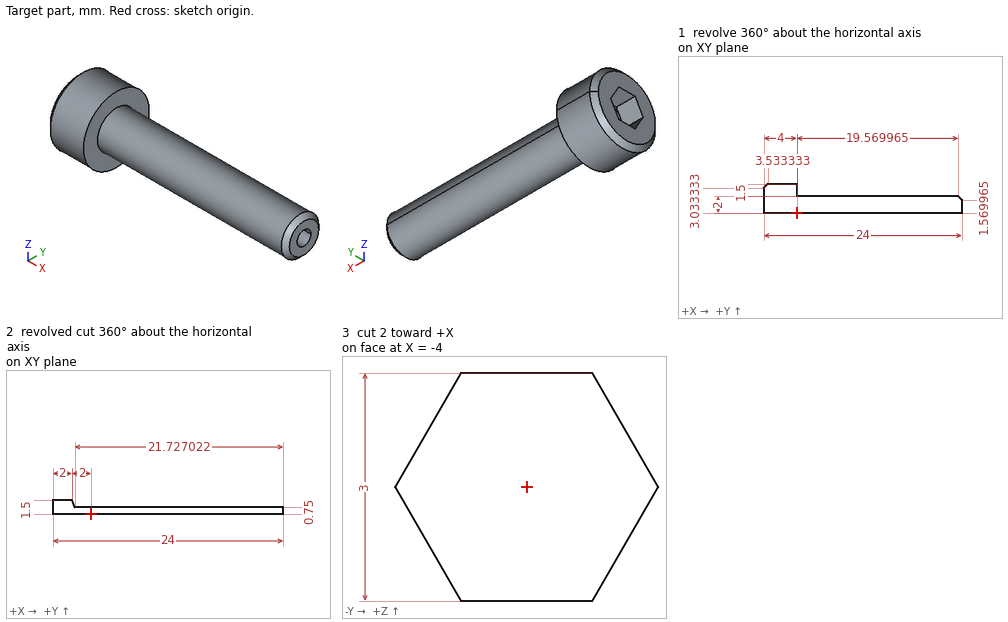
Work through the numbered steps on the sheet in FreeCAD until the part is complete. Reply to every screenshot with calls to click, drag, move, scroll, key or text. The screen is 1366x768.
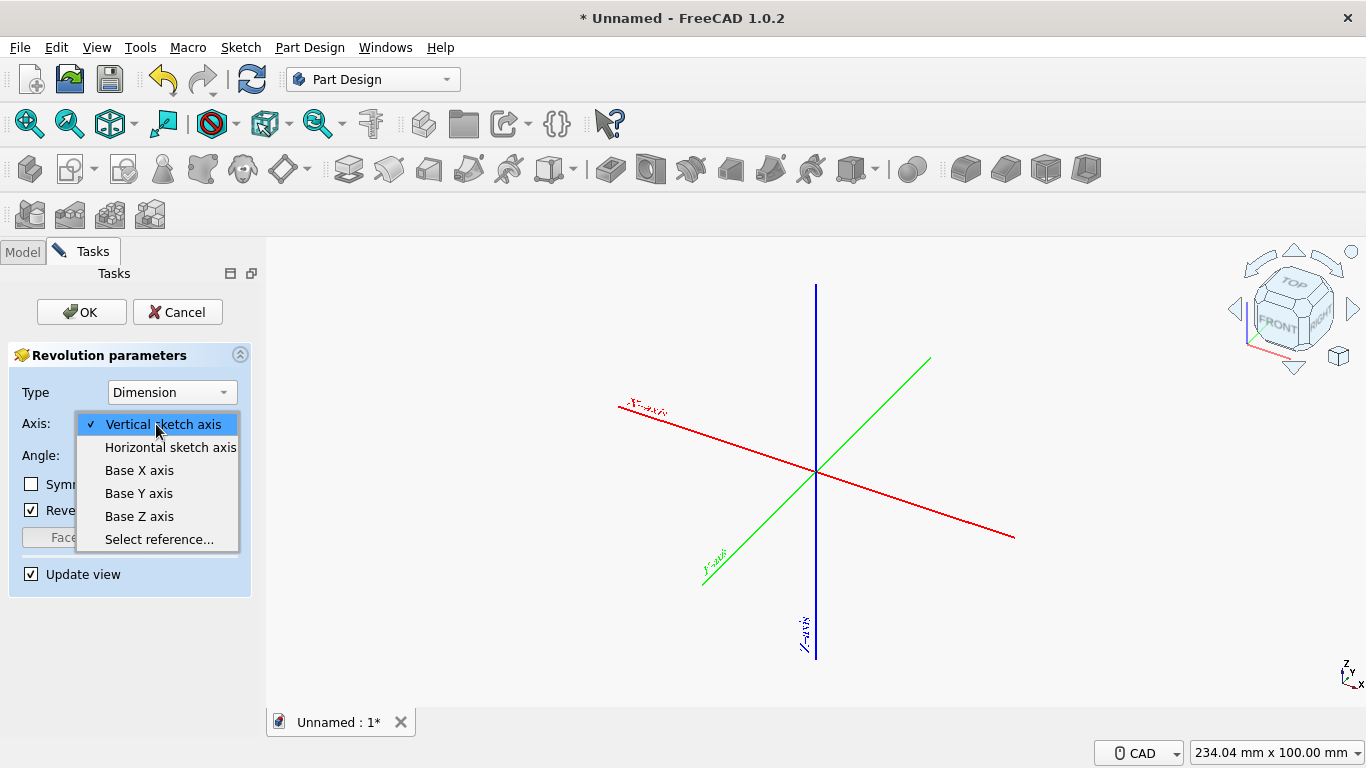
click(156, 448)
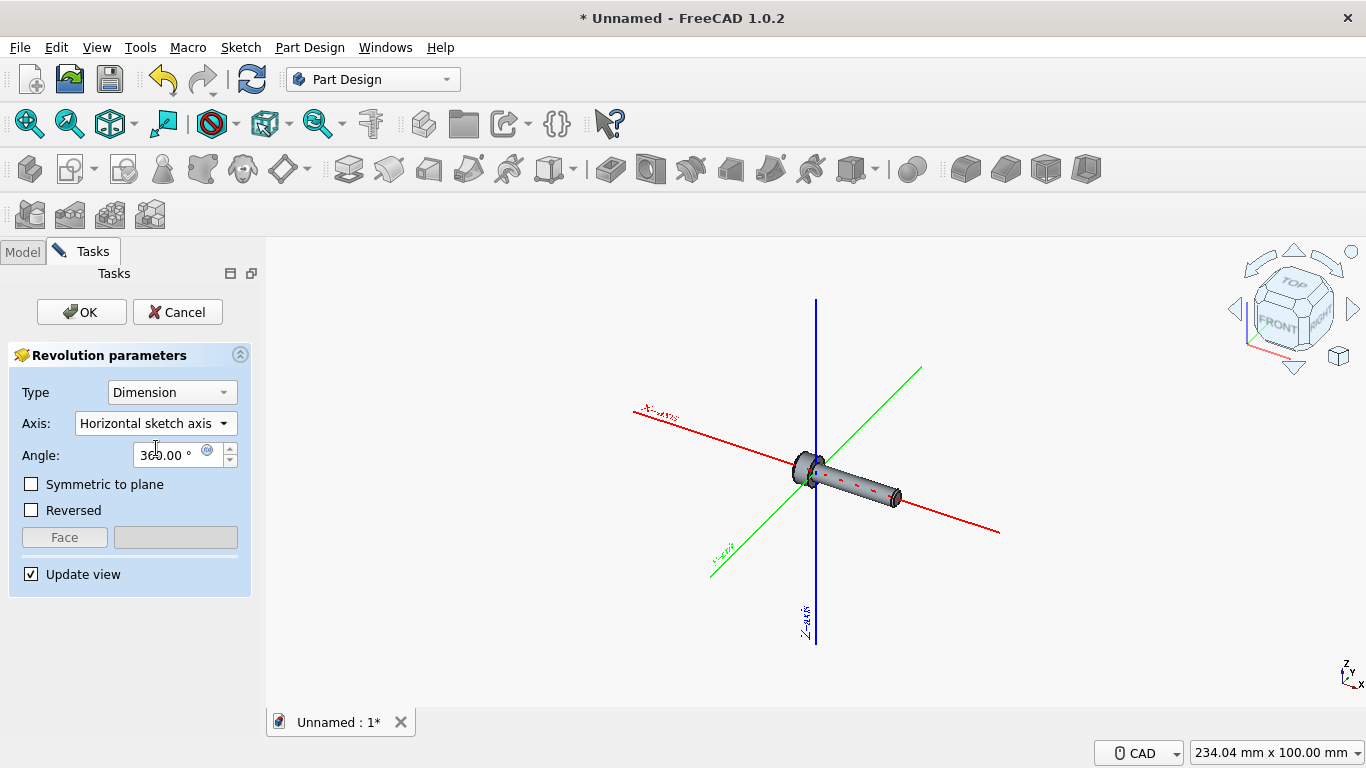
click(82, 312)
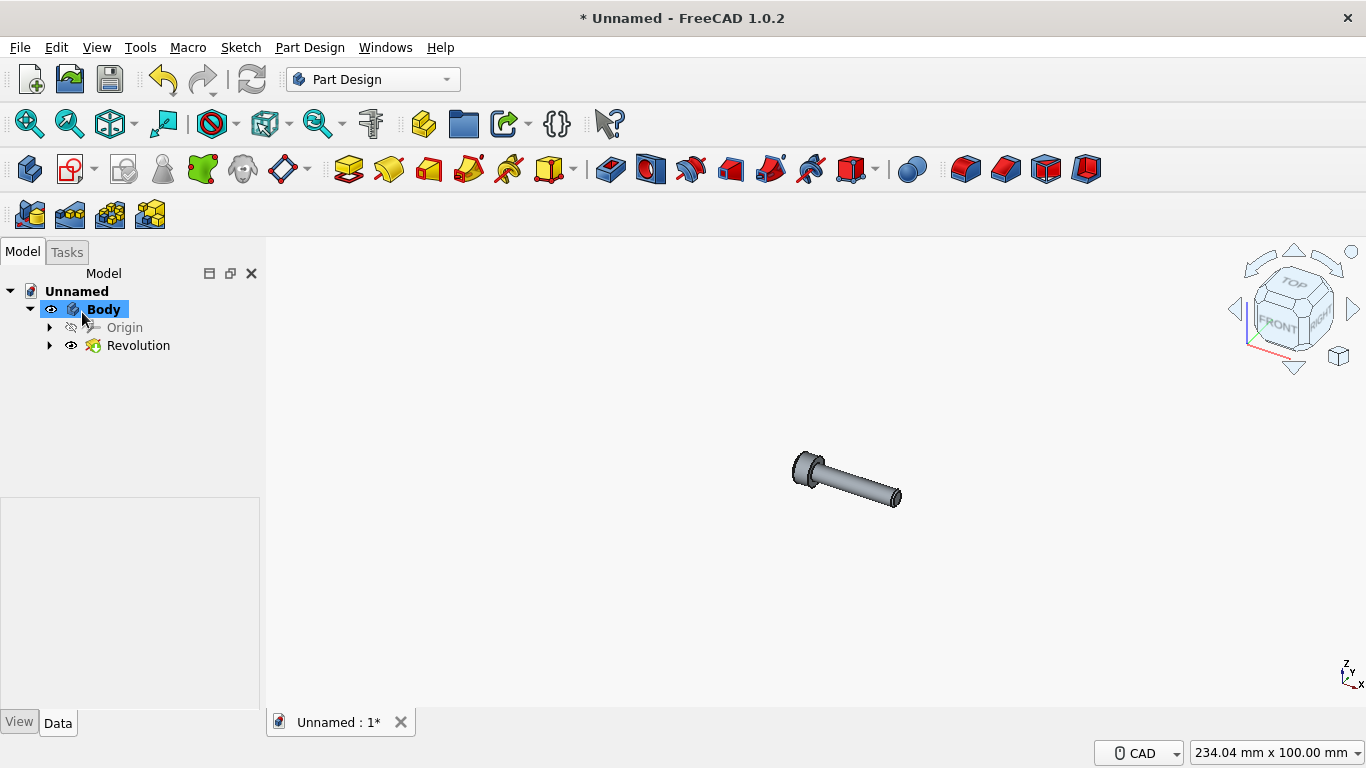
click(30, 124)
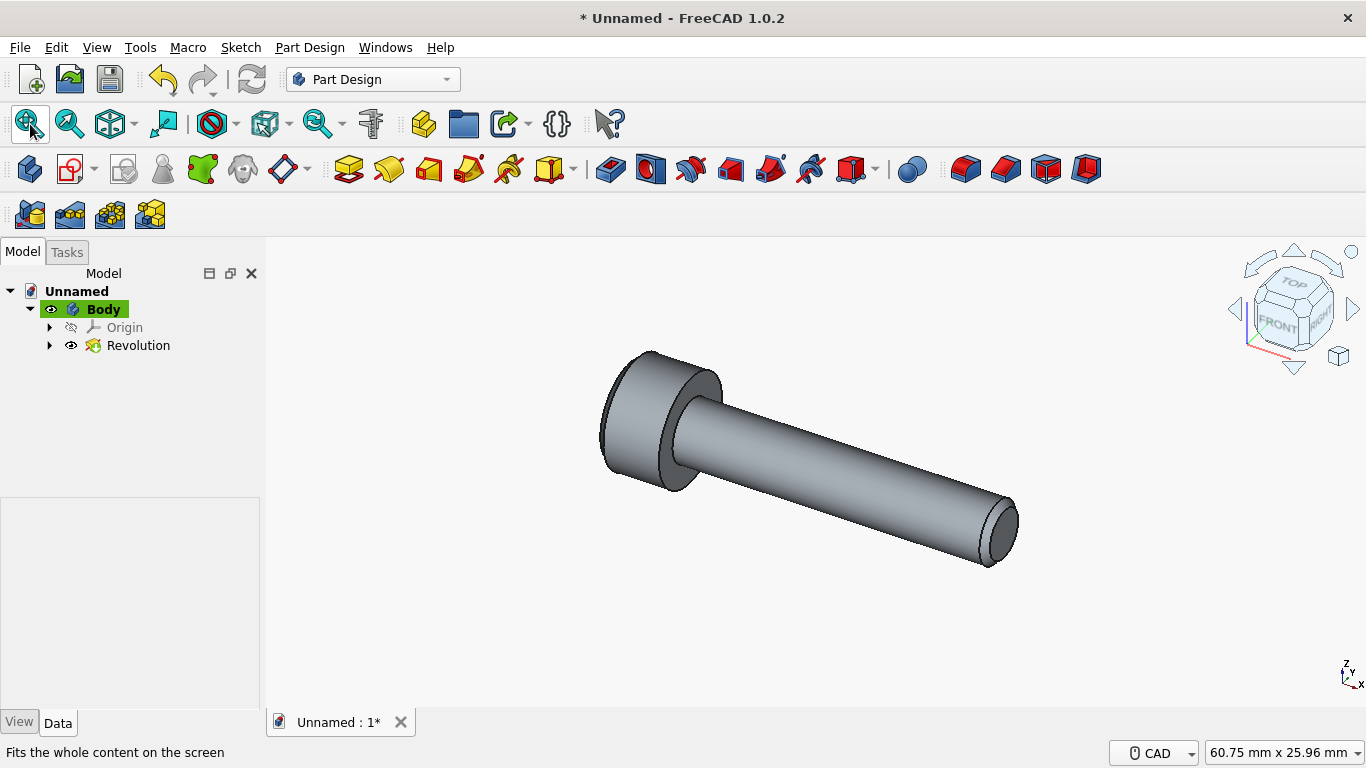
click(70, 170)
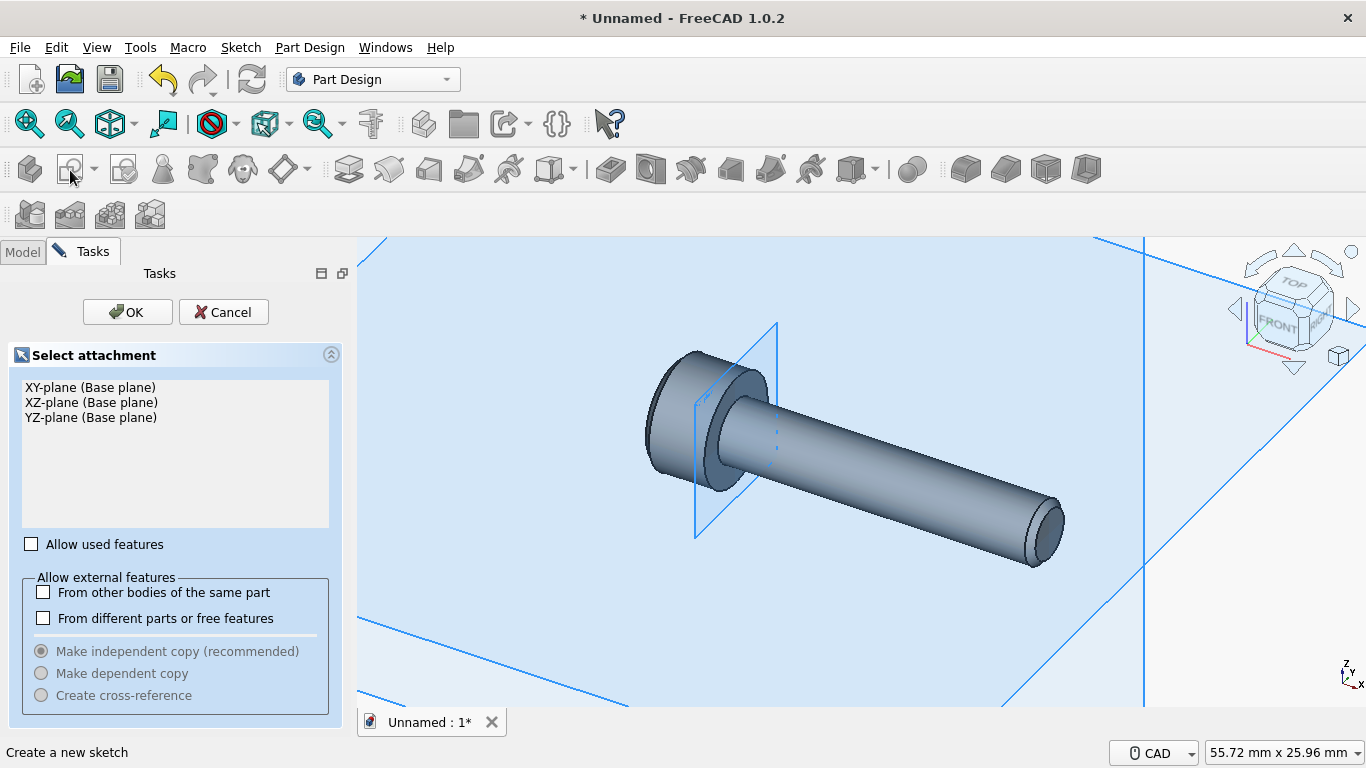
click(82, 388)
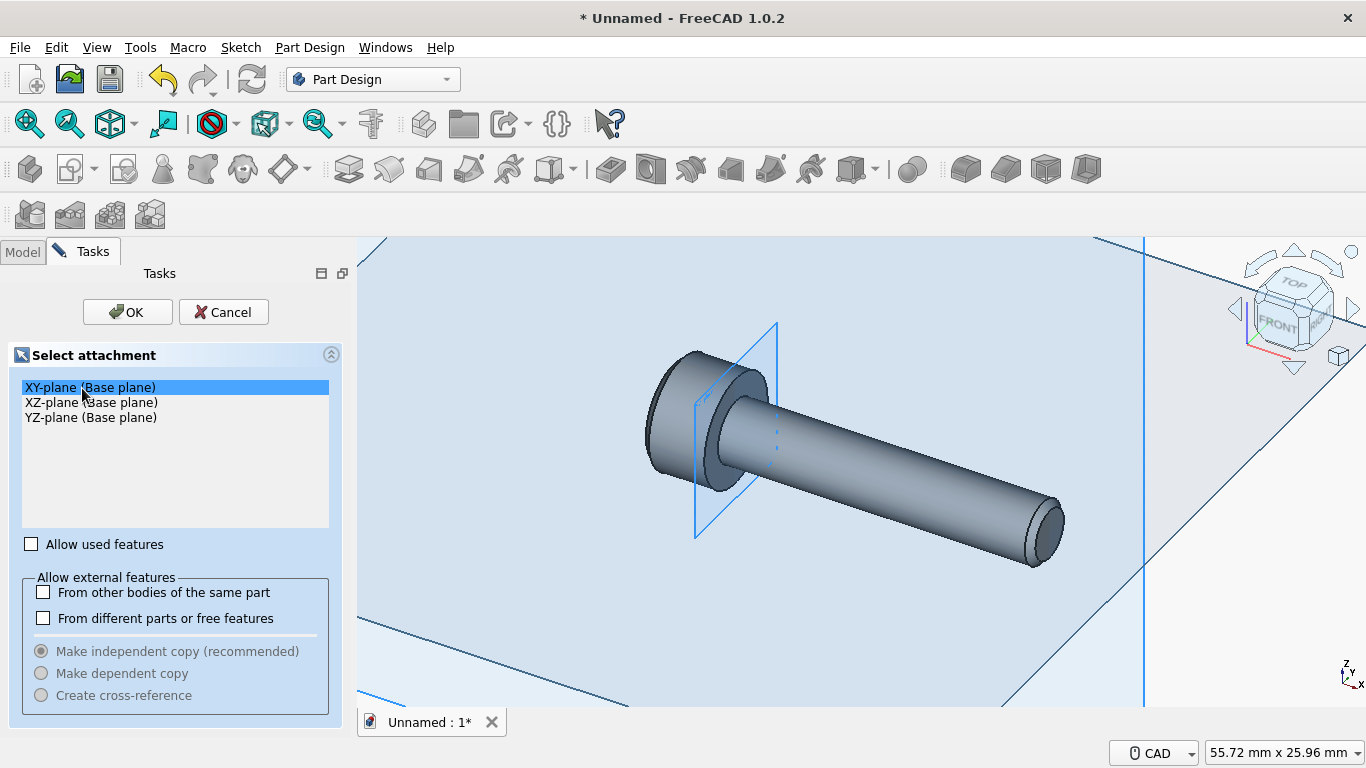
click(128, 312)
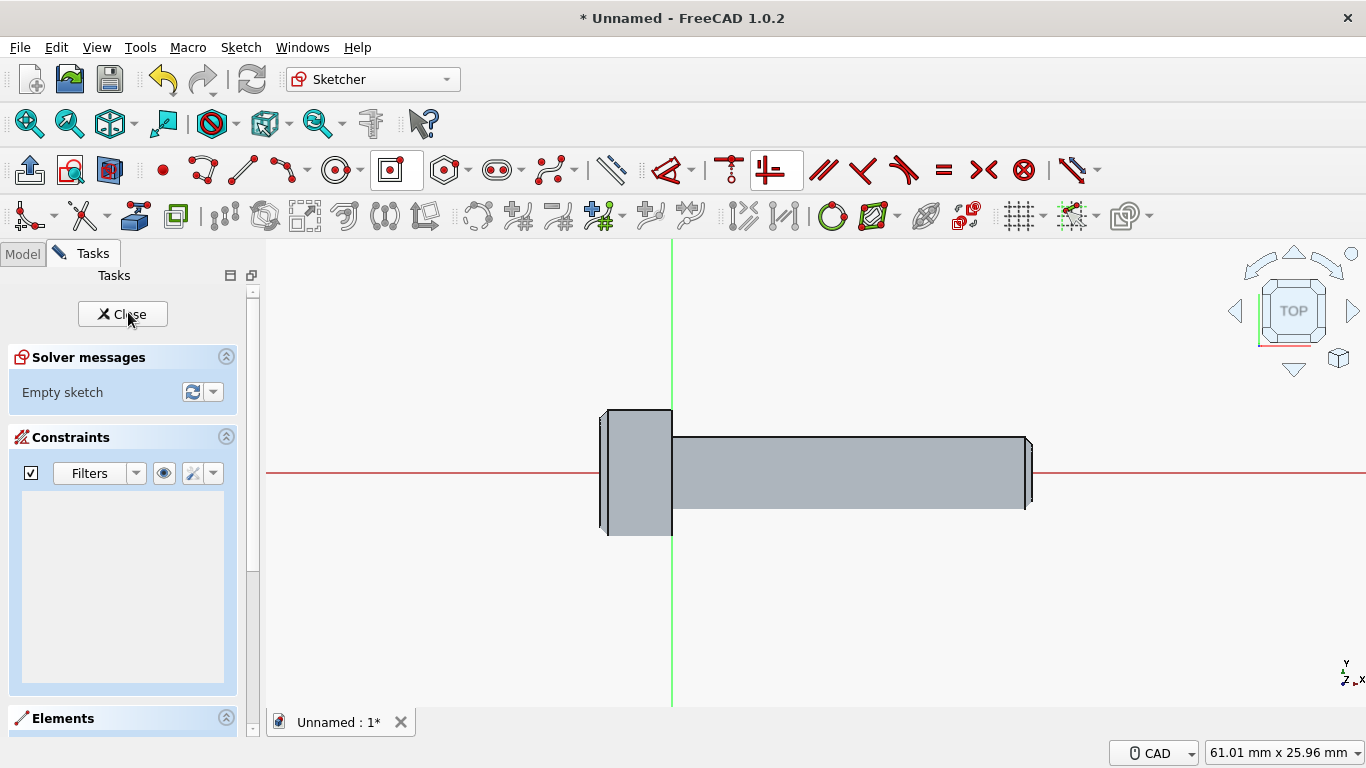
click(110, 170)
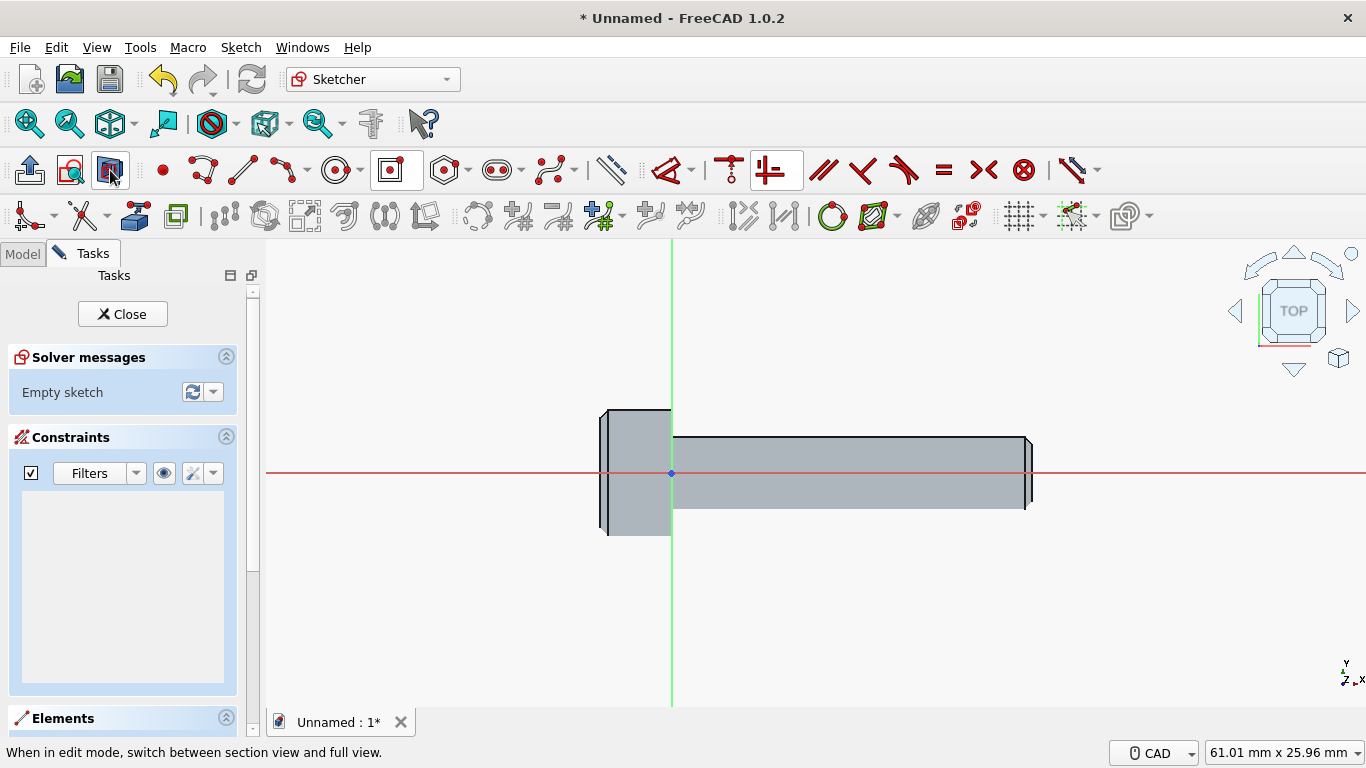
scroll(955, 432, up, 2)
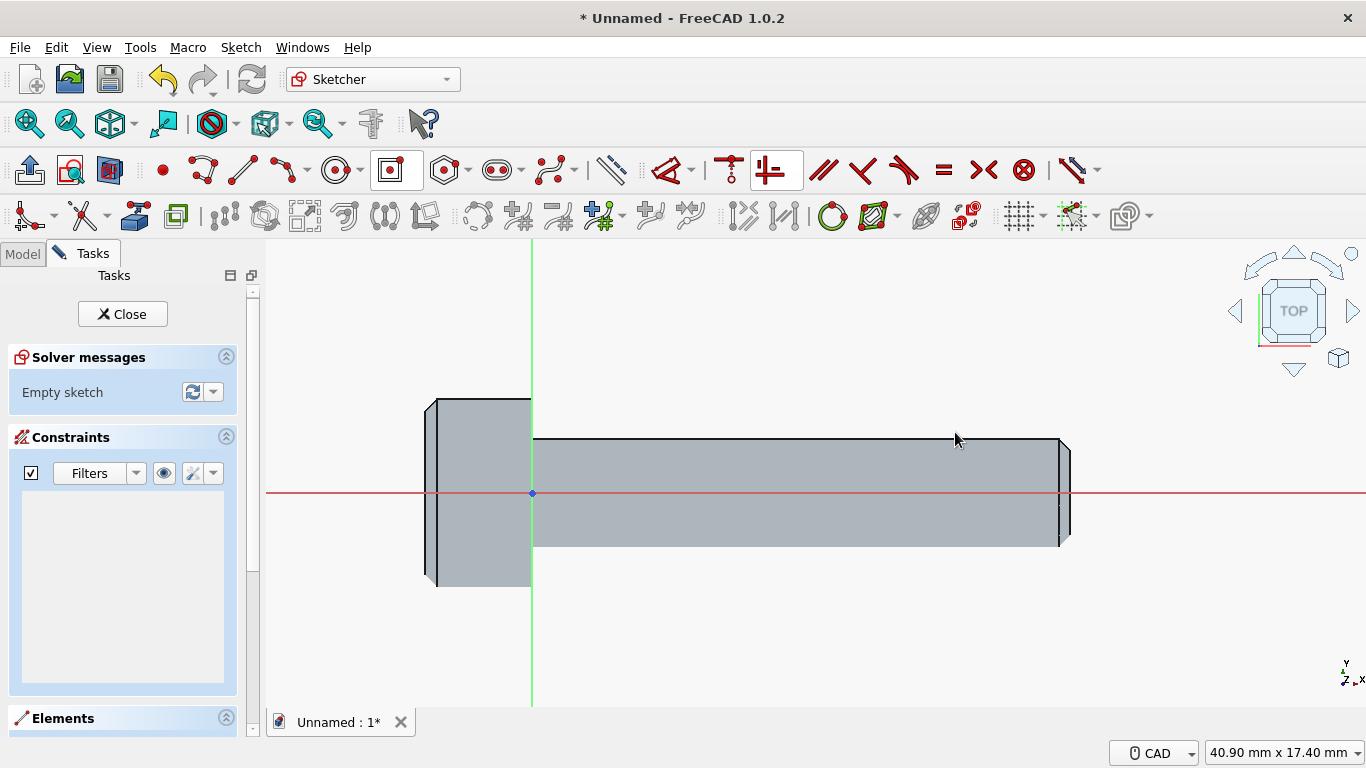
click(204, 170)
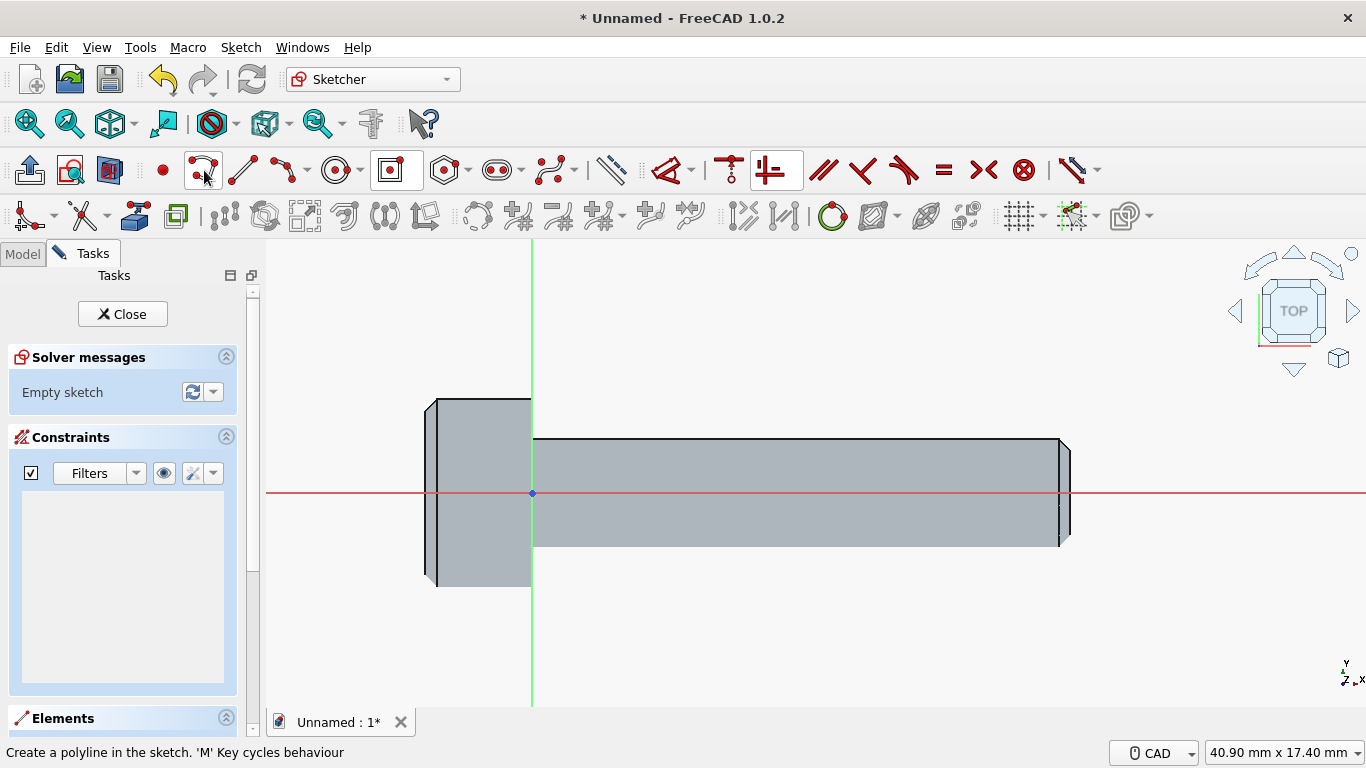
click(486, 473)
click(478, 453)
click(425, 453)
click(425, 493)
click(1070, 484)
click(1070, 473)